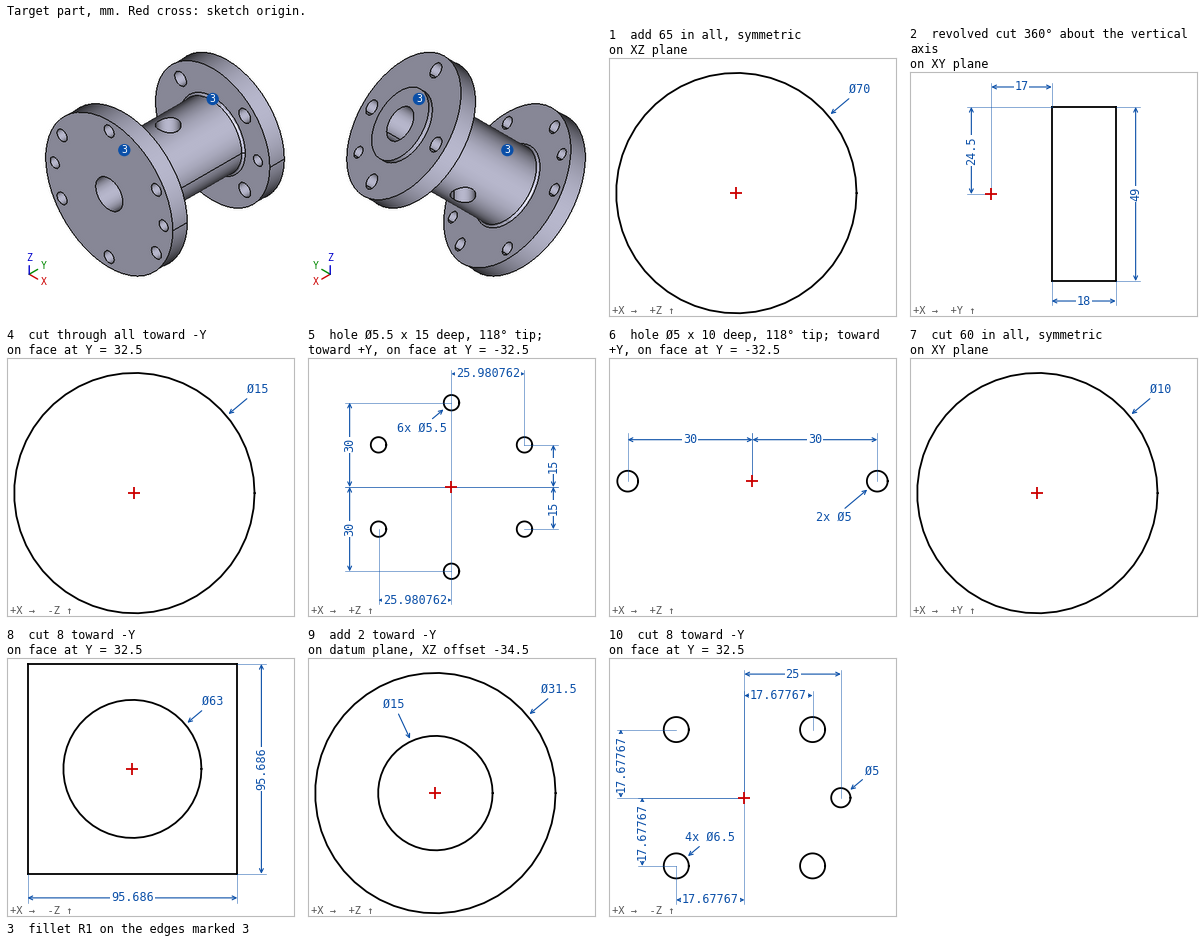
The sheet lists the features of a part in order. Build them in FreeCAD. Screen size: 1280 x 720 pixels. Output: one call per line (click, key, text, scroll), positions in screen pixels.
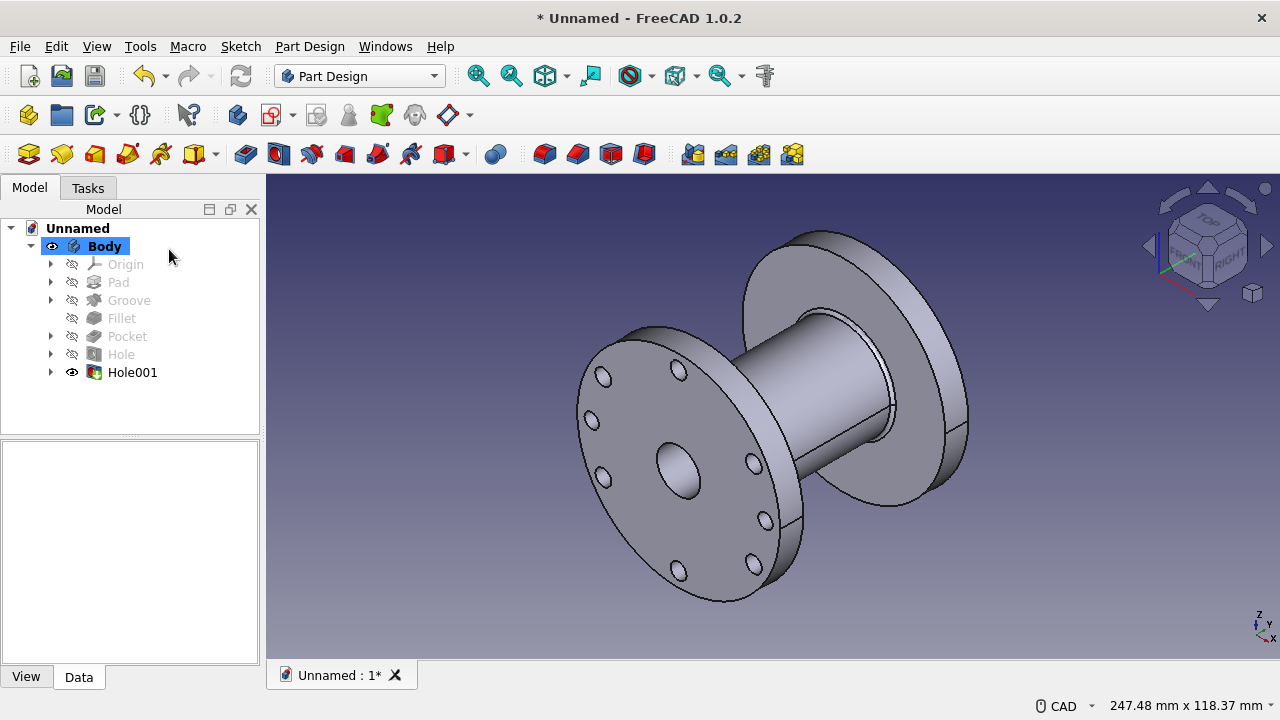
click(270, 116)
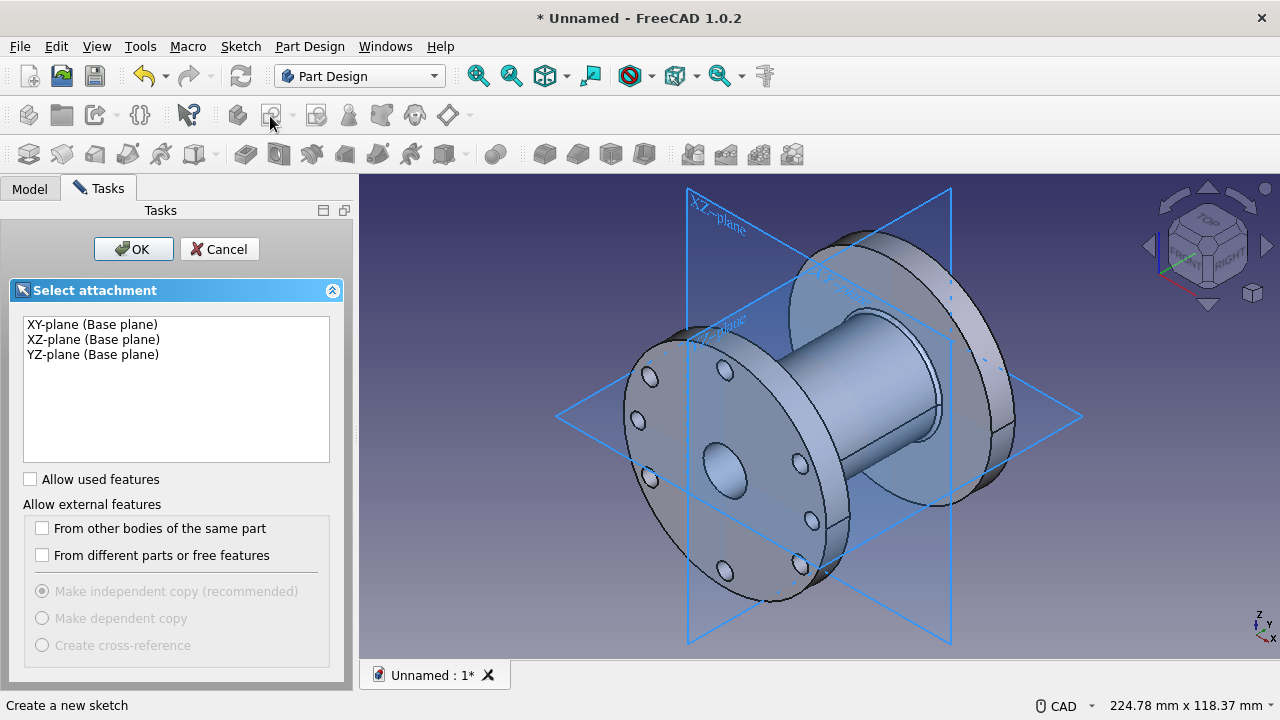
click(84, 324)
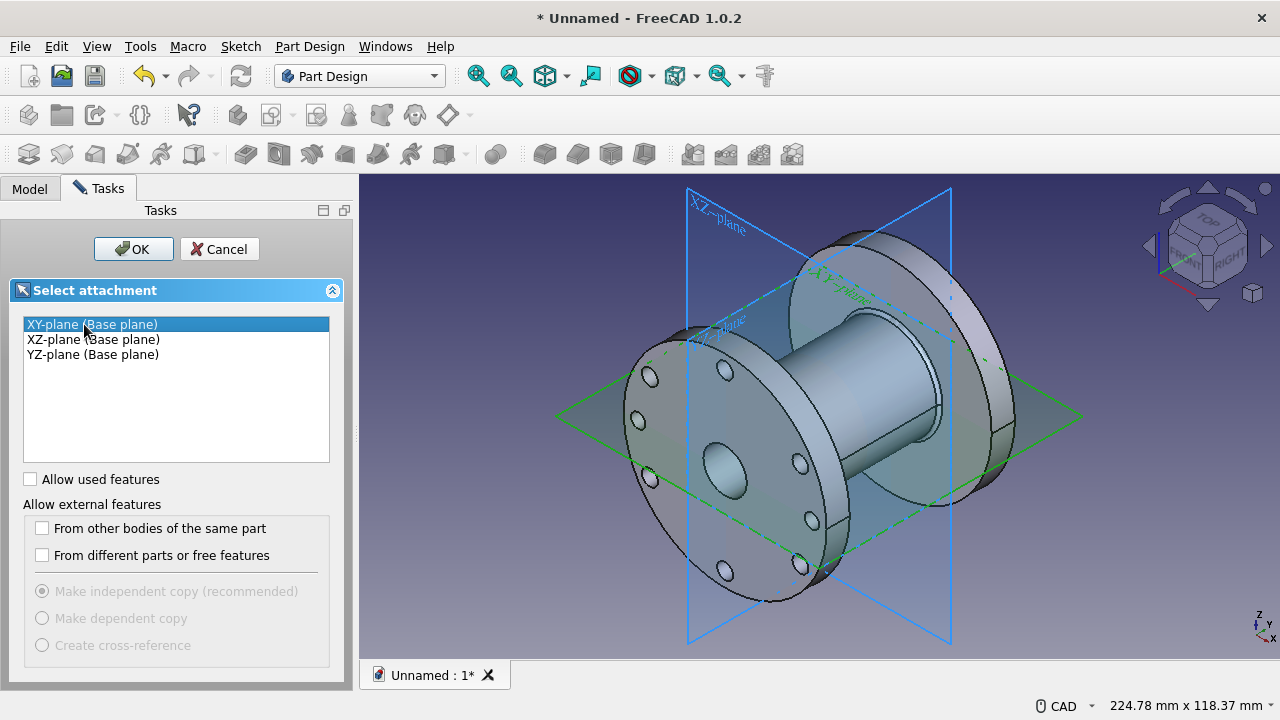
click(134, 249)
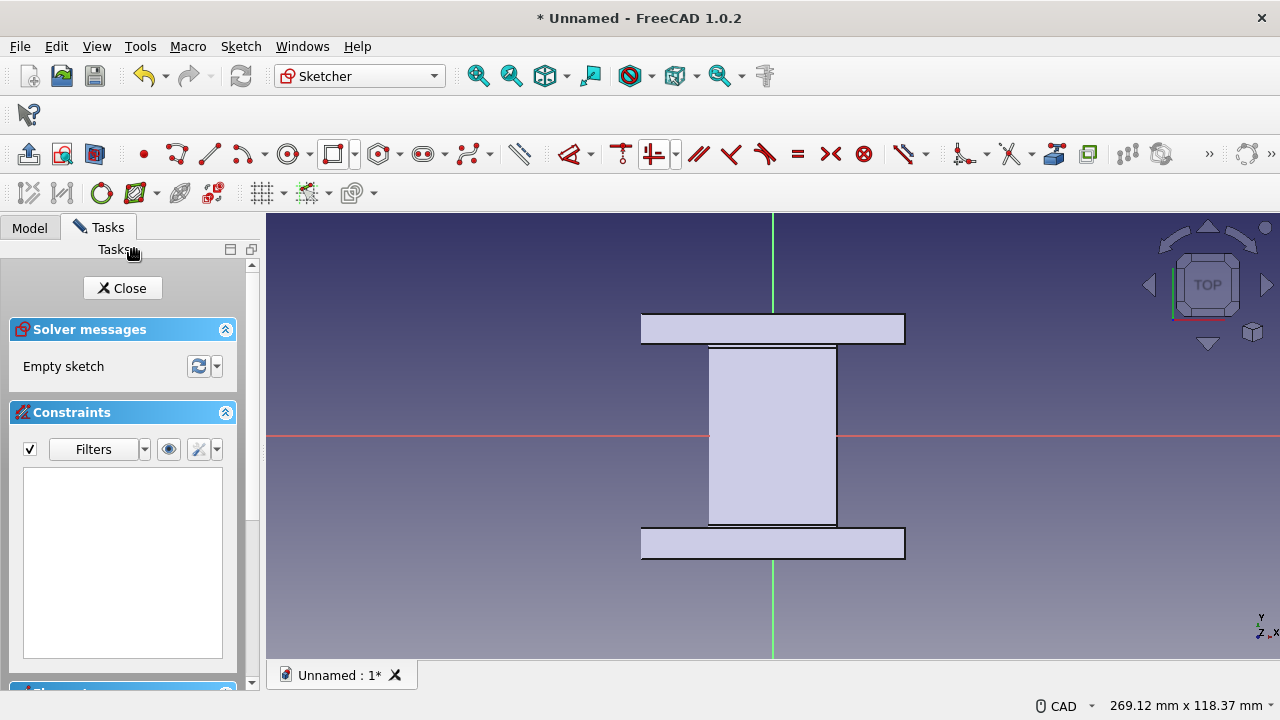
click(95, 154)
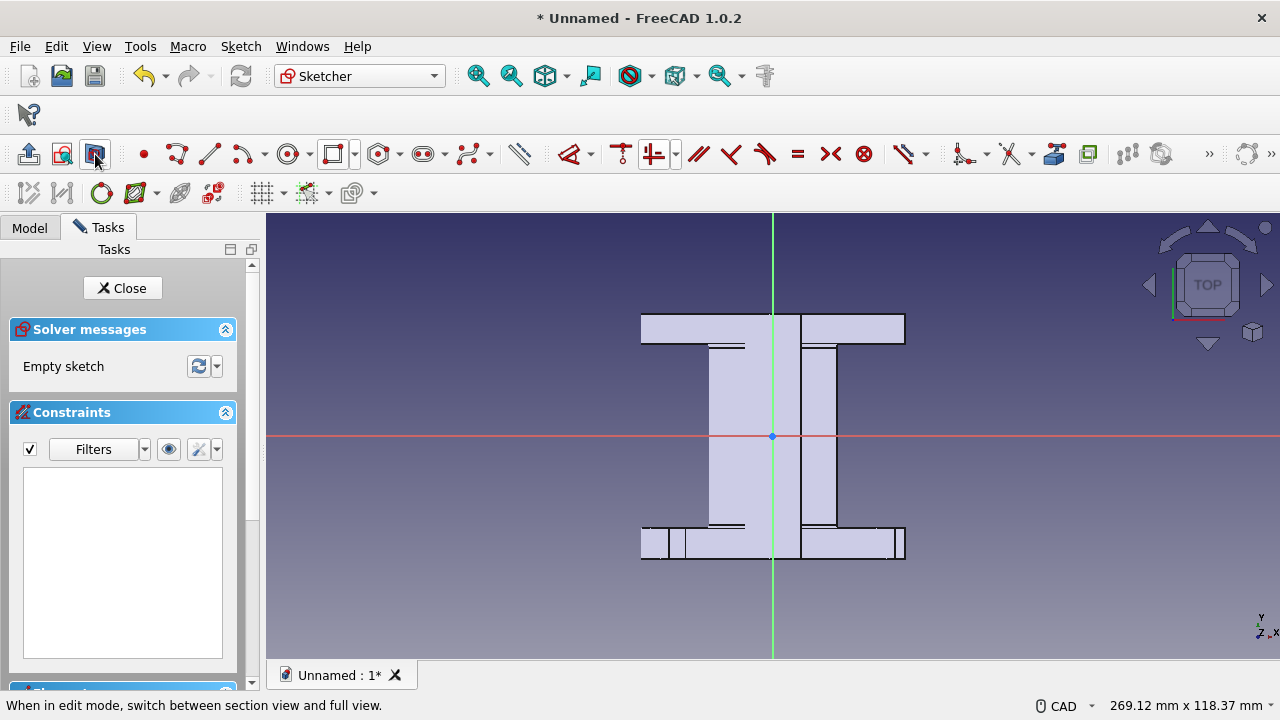
scroll(783, 436, up, 10)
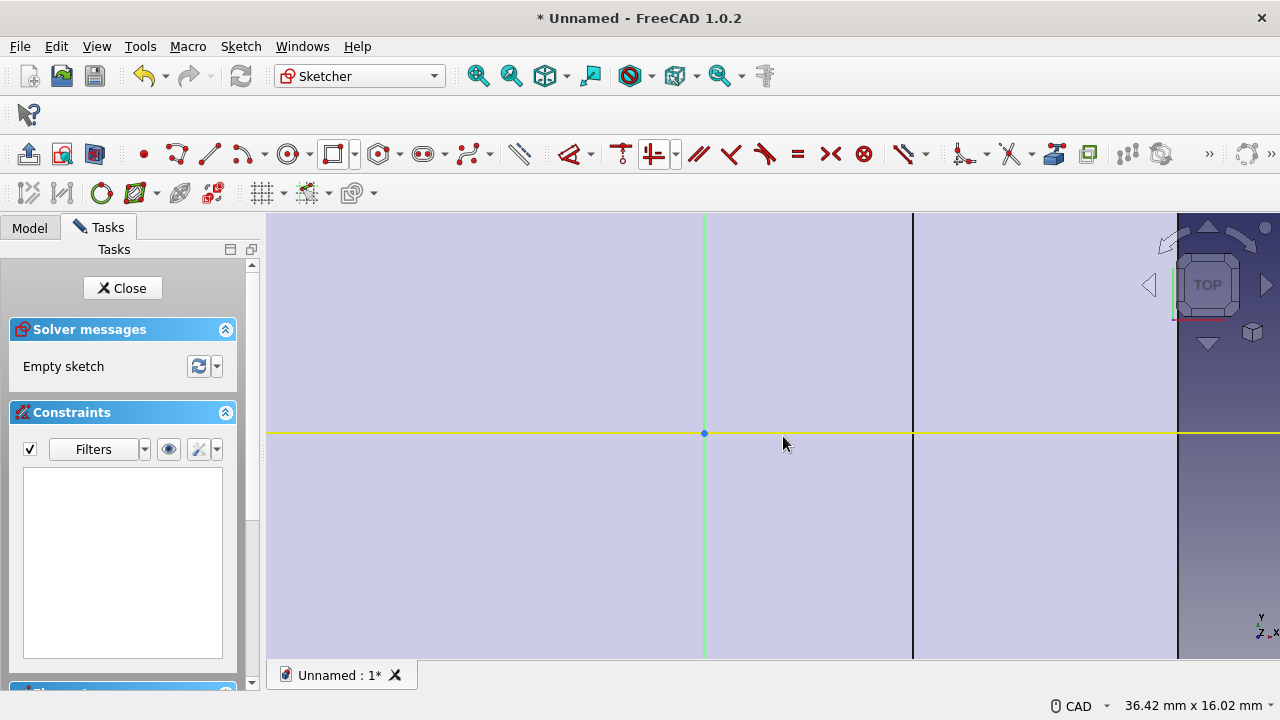
click(288, 154)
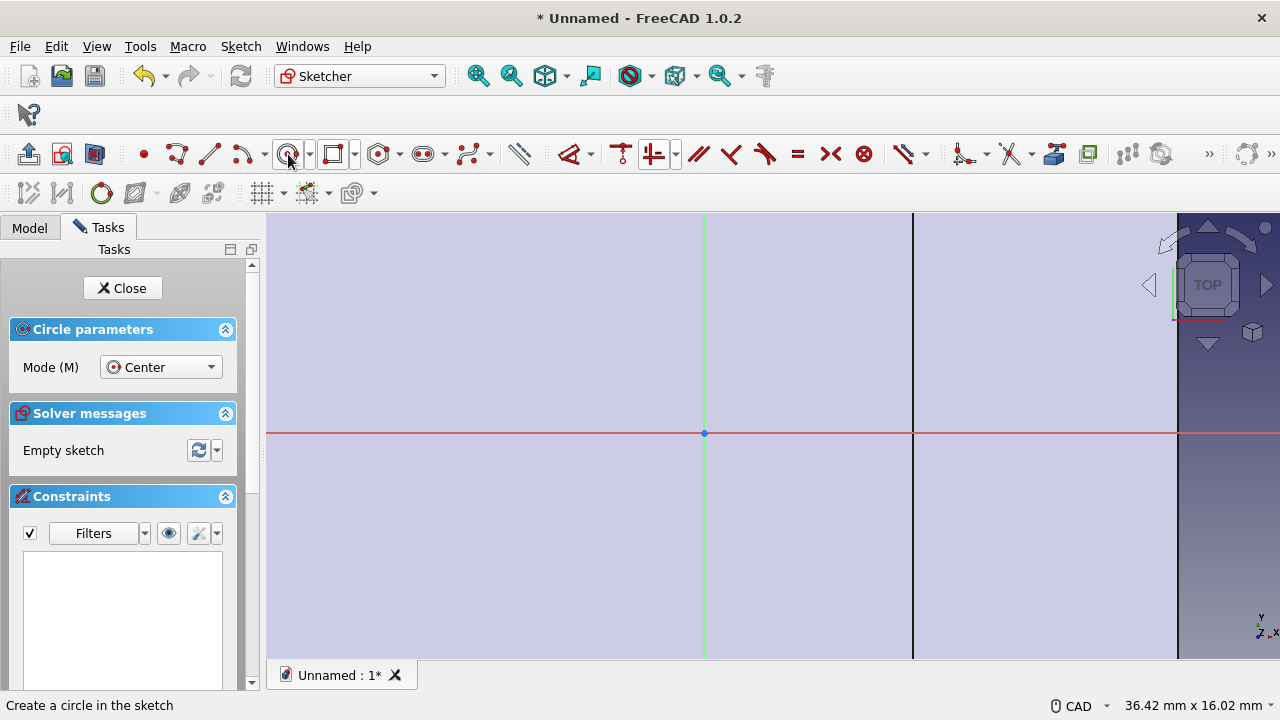
click(704, 433)
move(803, 335)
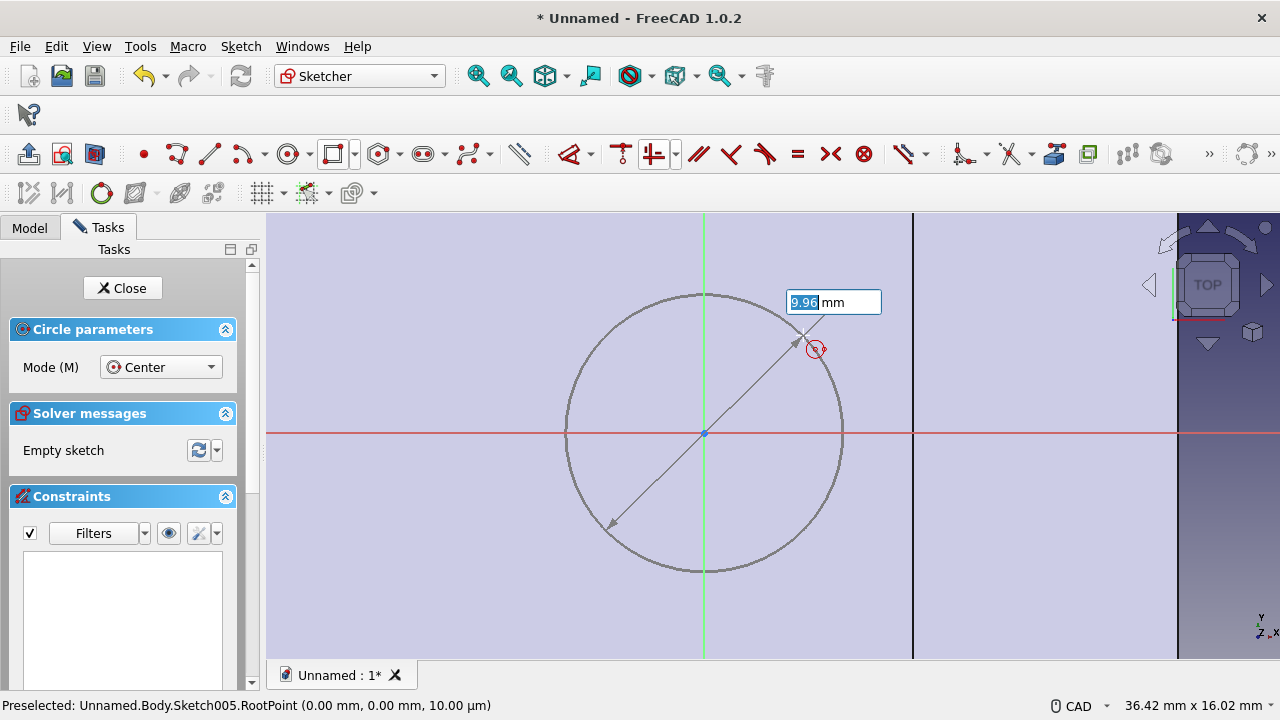
text(10)
key(Return)
key(Escape)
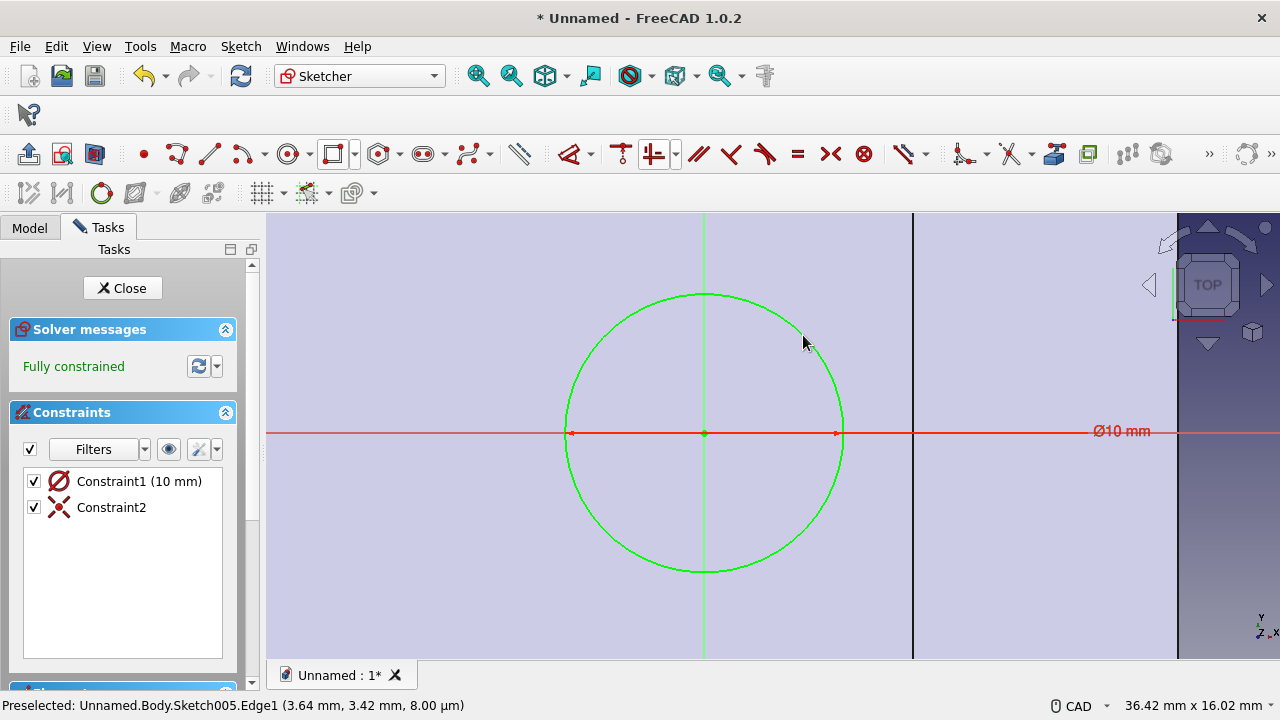
click(123, 288)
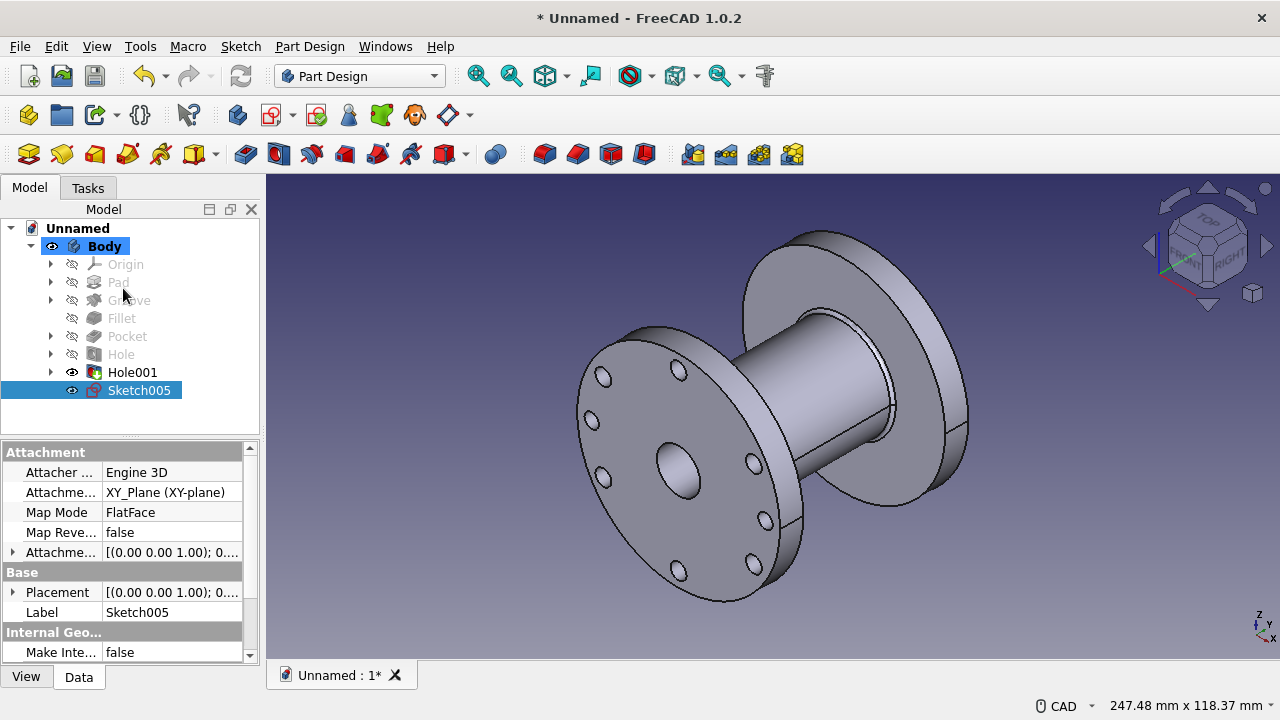
click(246, 154)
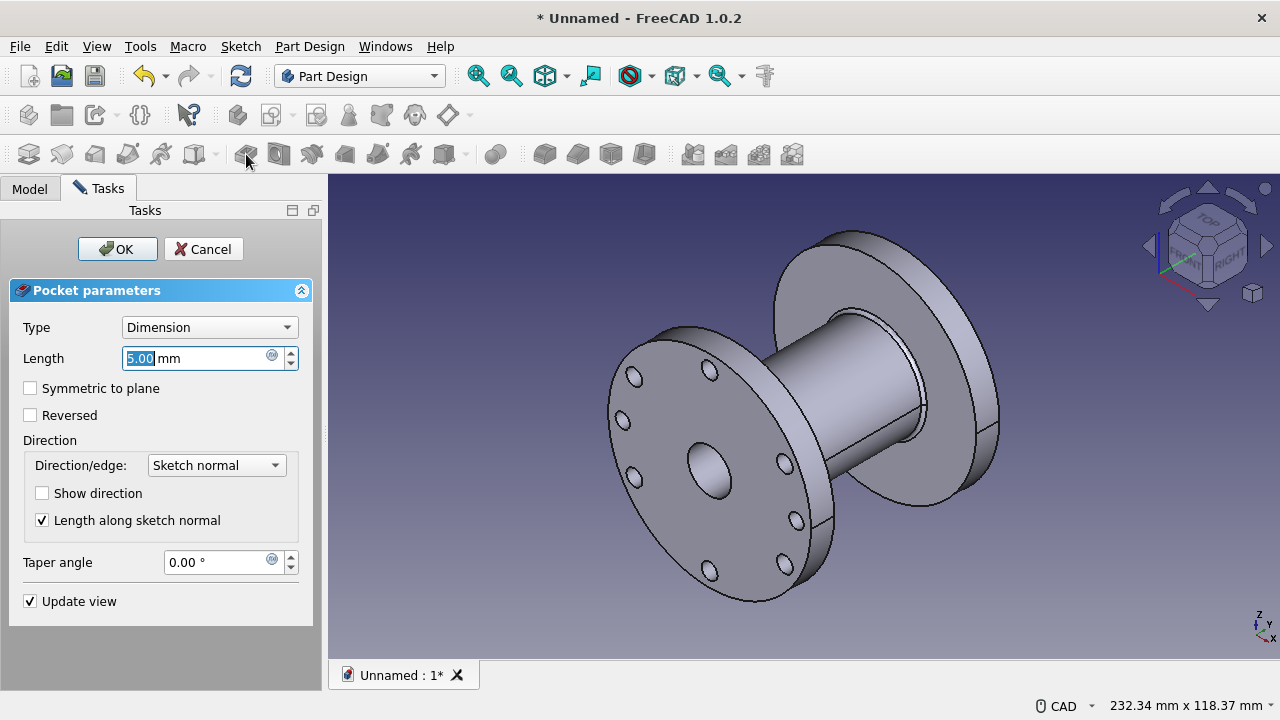
text(60)
key(Tab)